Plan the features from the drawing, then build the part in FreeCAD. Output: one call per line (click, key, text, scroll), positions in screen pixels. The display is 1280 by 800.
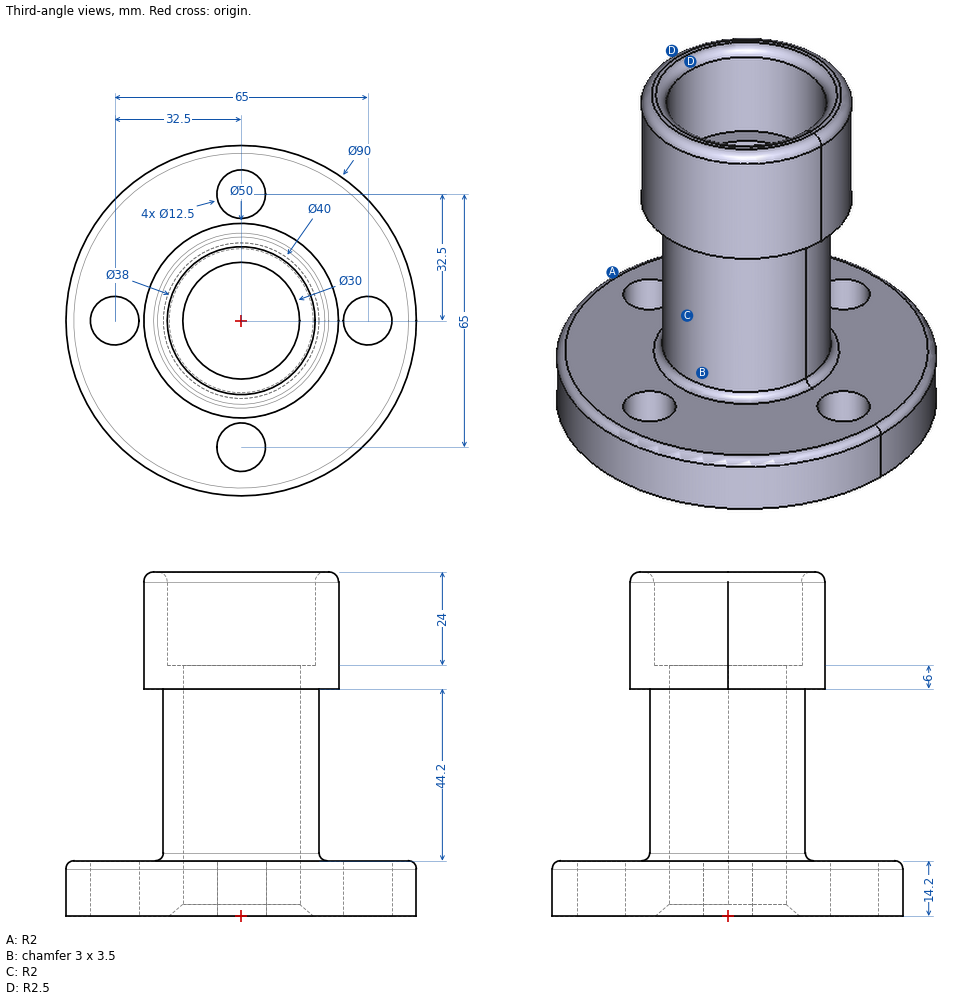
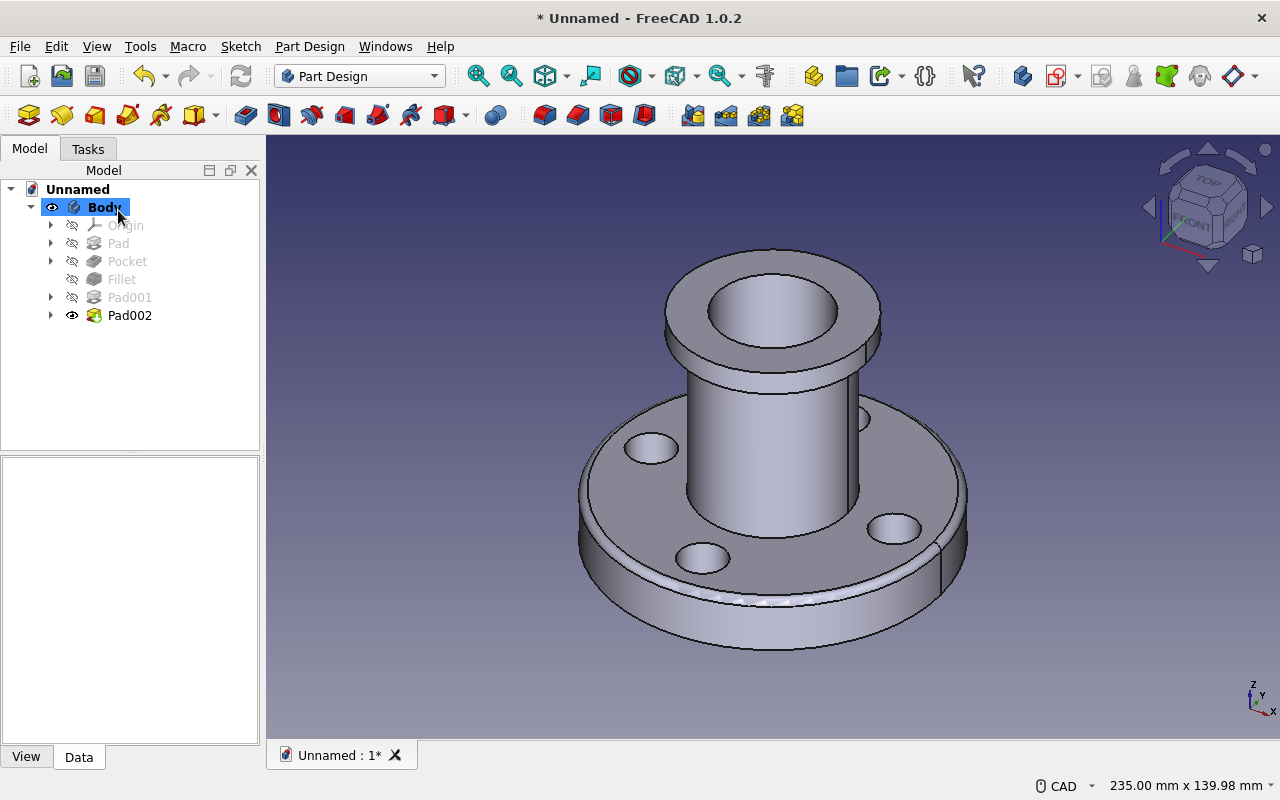
click(795, 359)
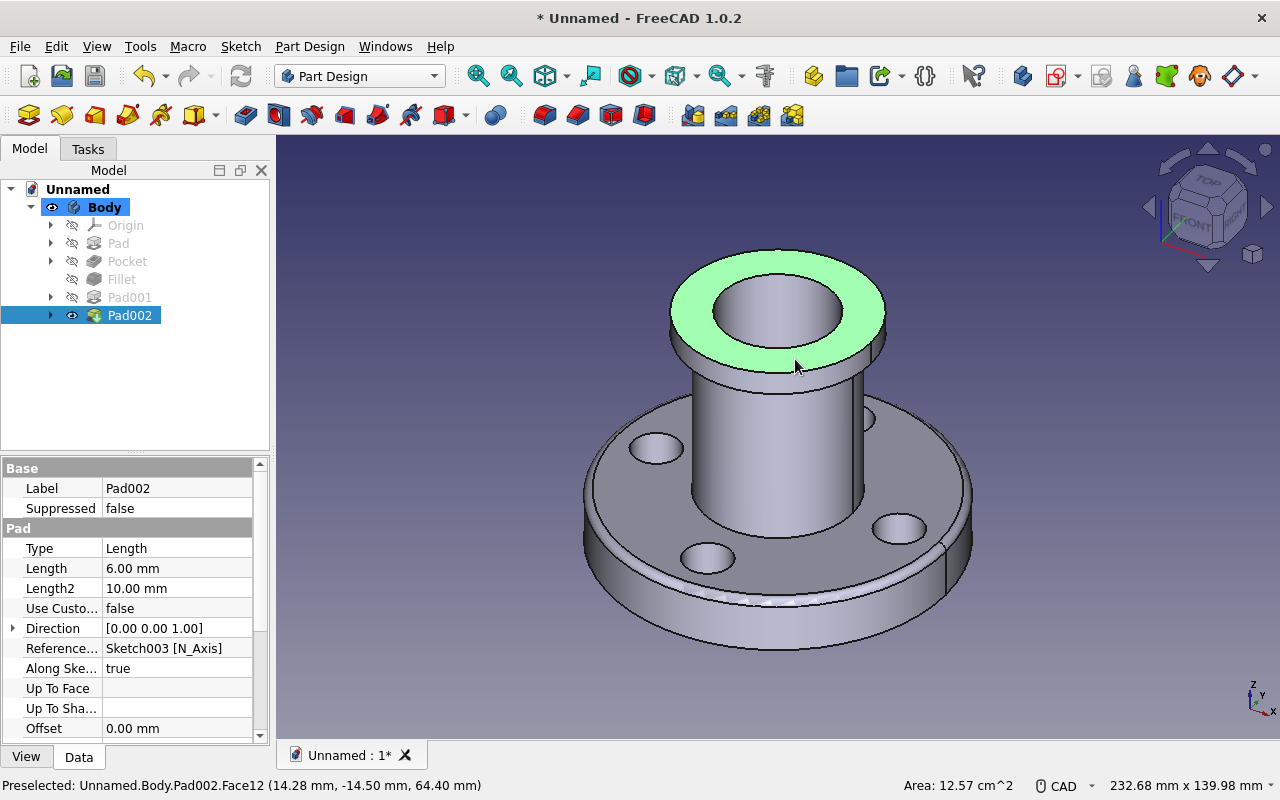
click(1056, 76)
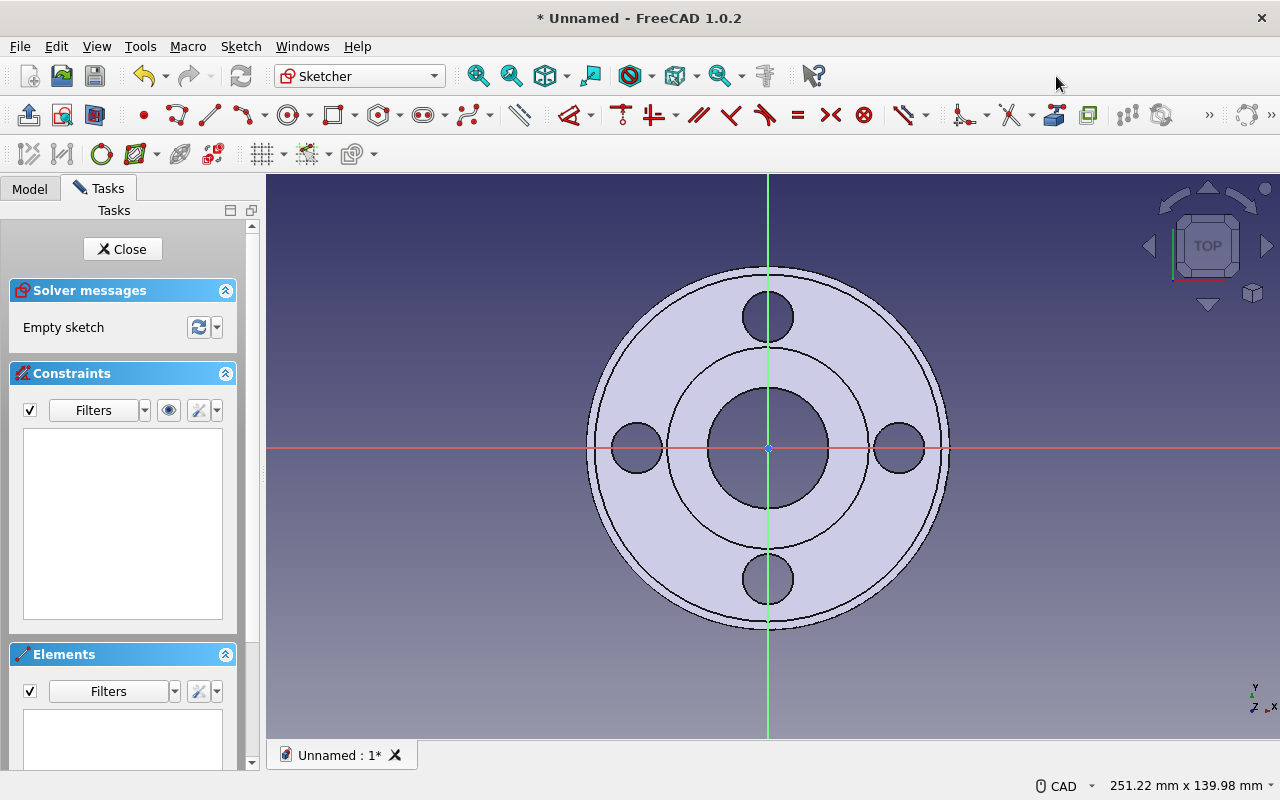
scroll(845, 438, up, 3)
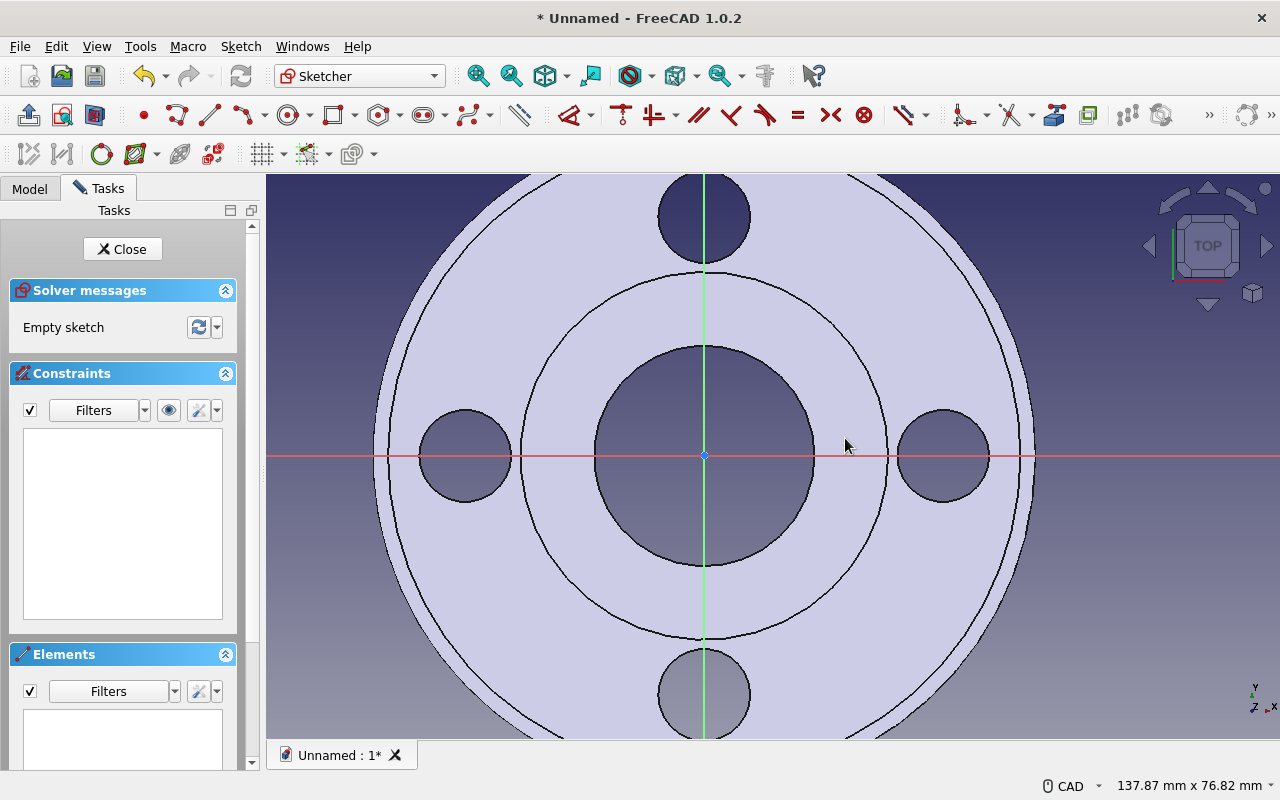
key(g)
key(c)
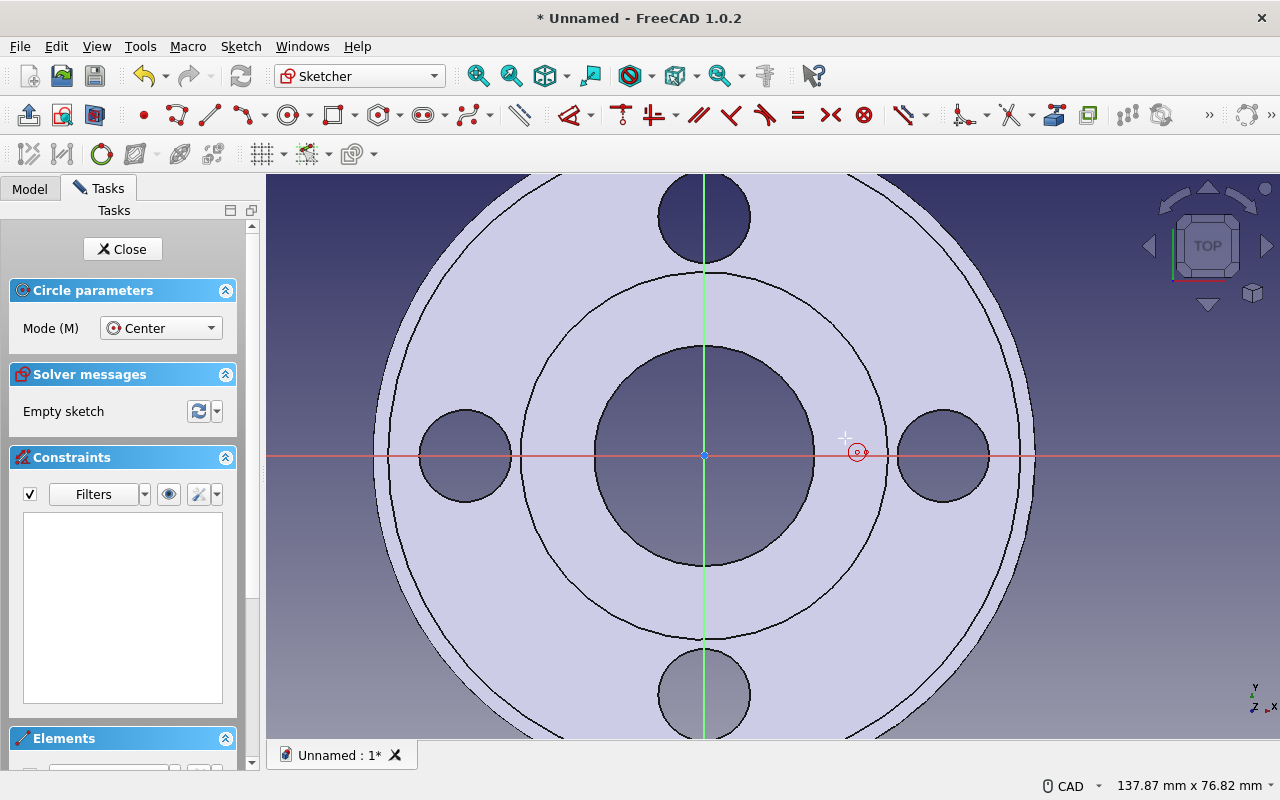
click(704, 456)
move(834, 326)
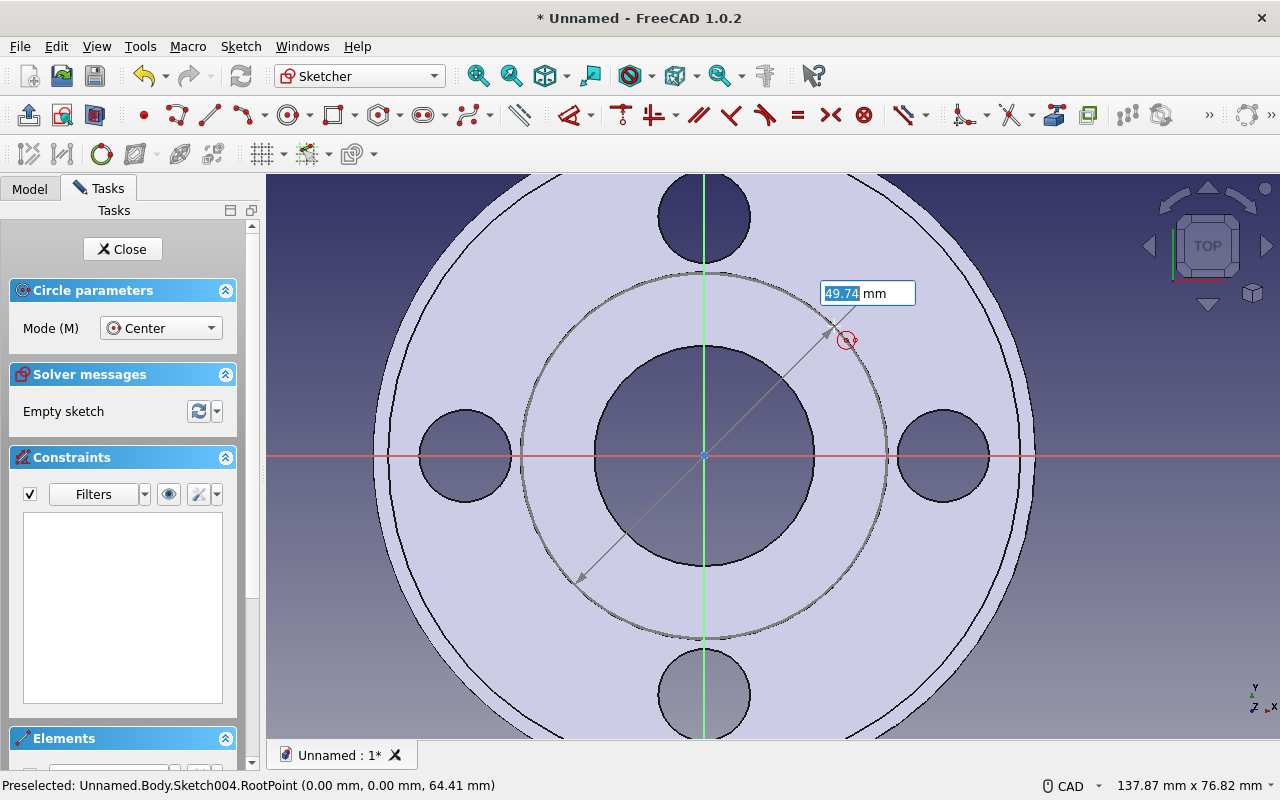
text(50)
key(Return)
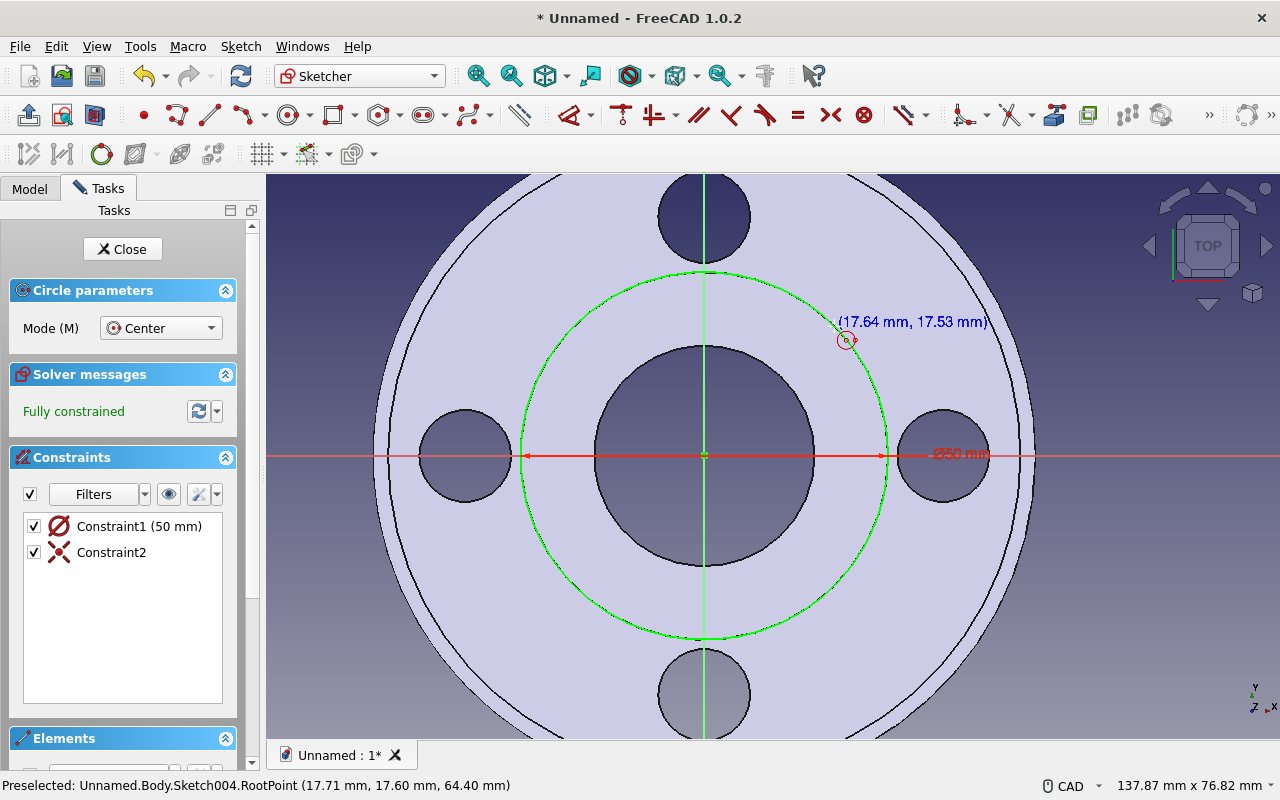
click(704, 456)
move(803, 357)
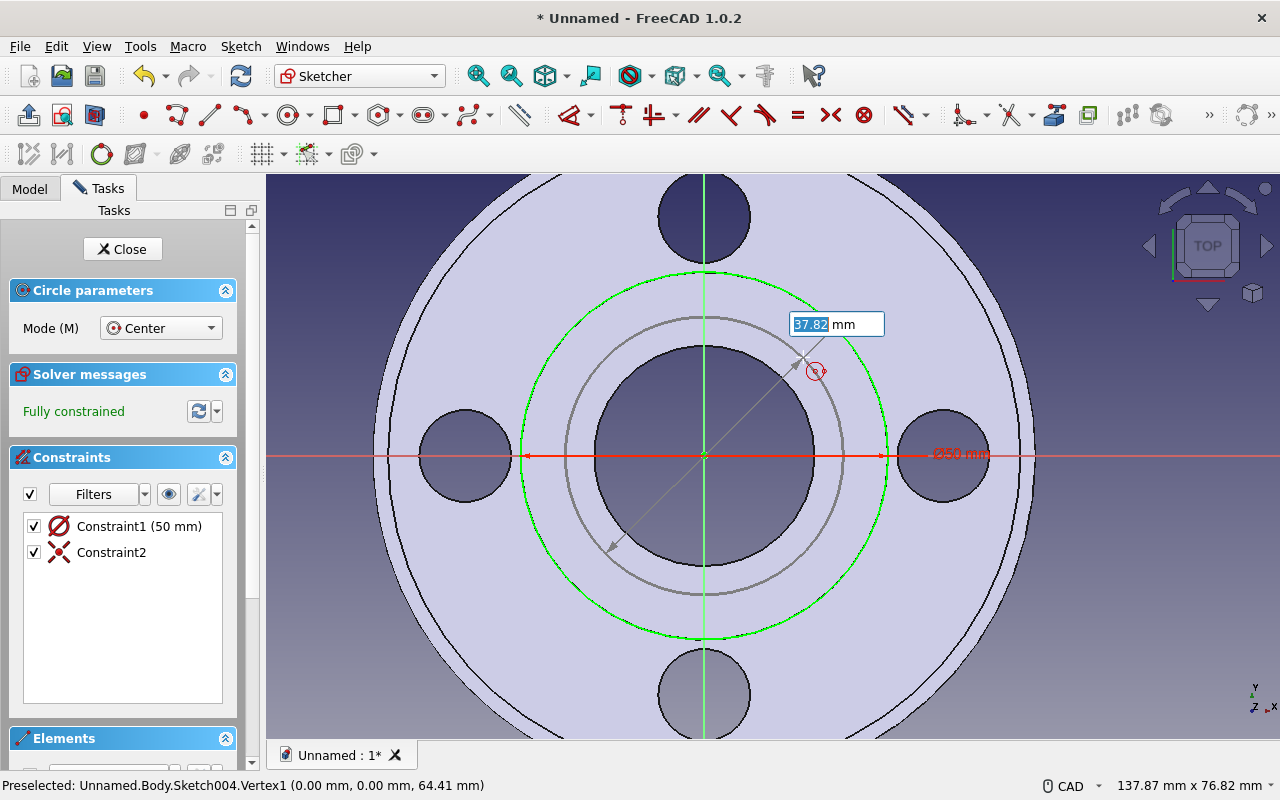
text(38)
key(Return)
key(Escape)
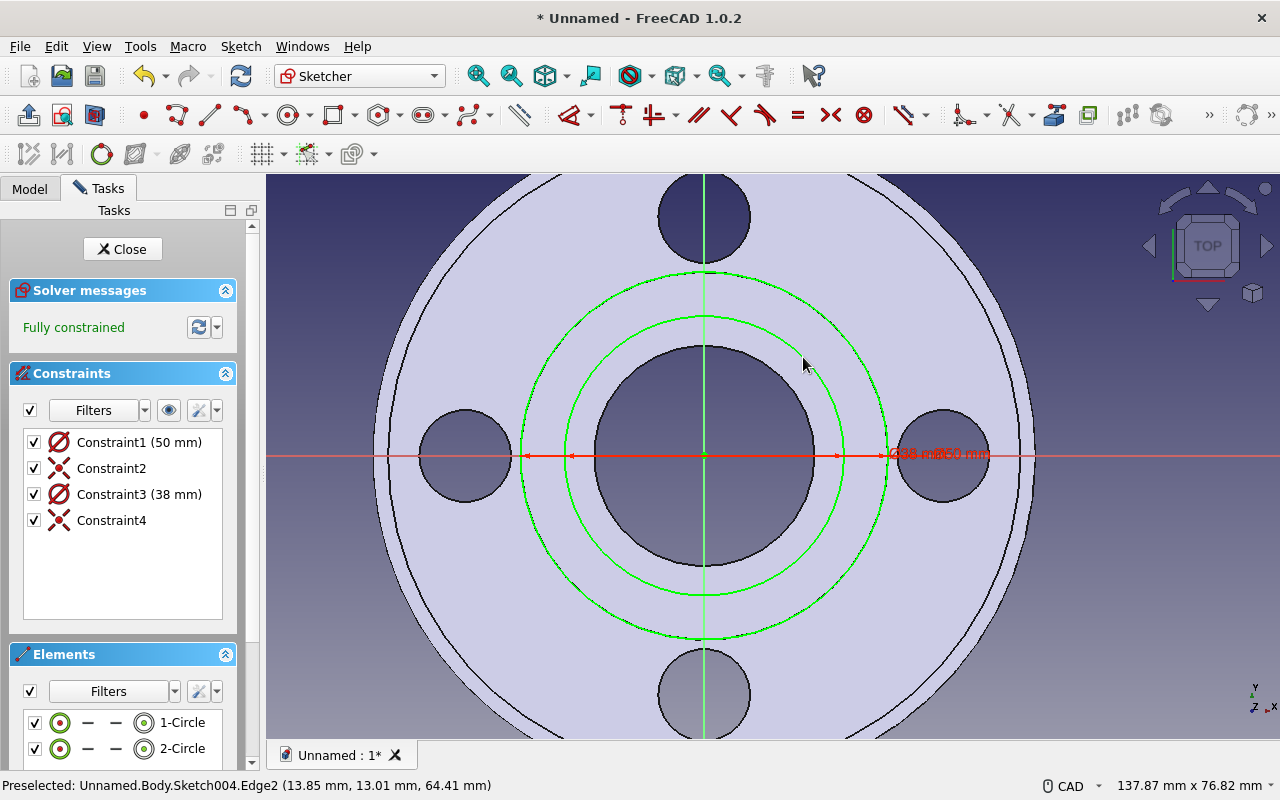
click(123, 249)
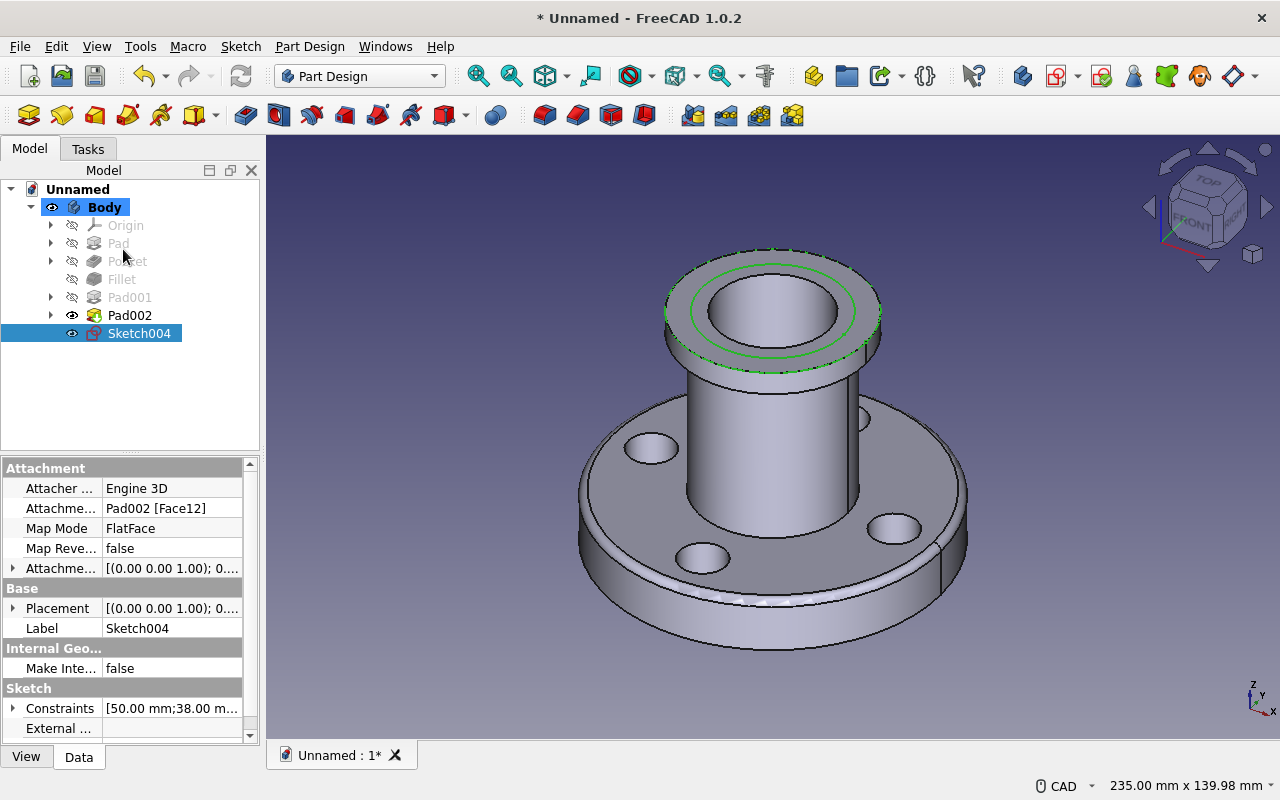
click(29, 116)